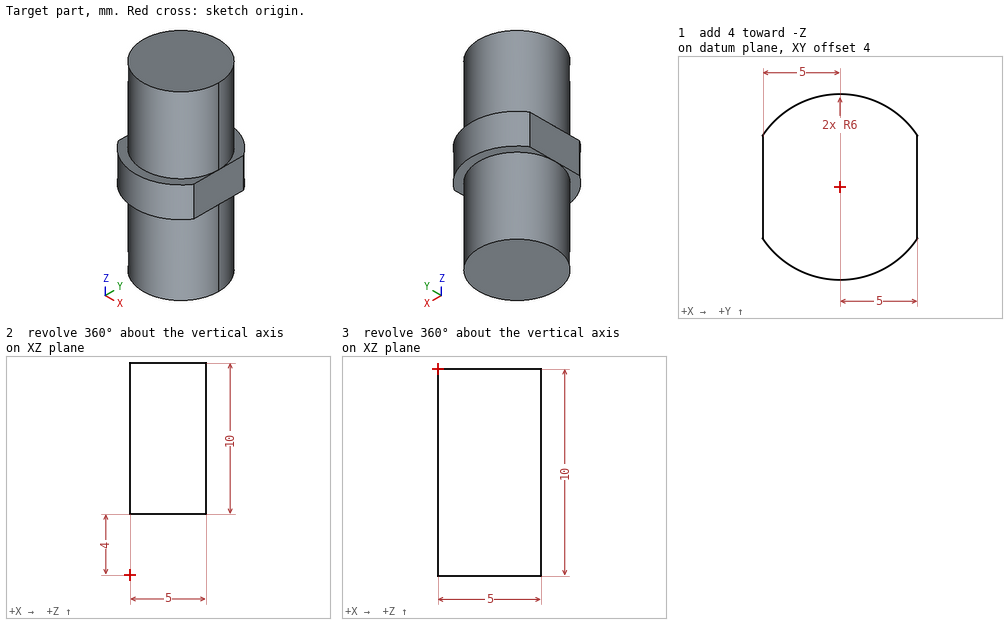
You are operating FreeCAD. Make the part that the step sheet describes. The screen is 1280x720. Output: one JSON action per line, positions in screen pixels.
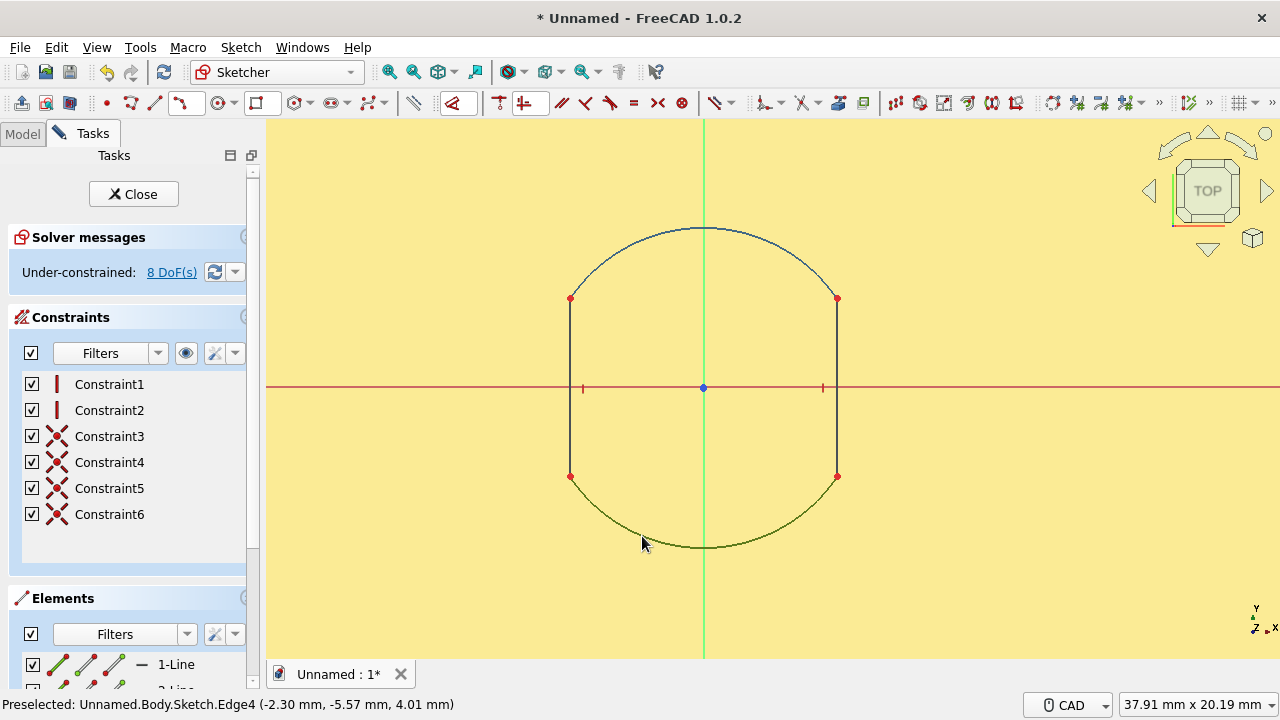
{"action": "left_click", "coordinate": [500, 104]}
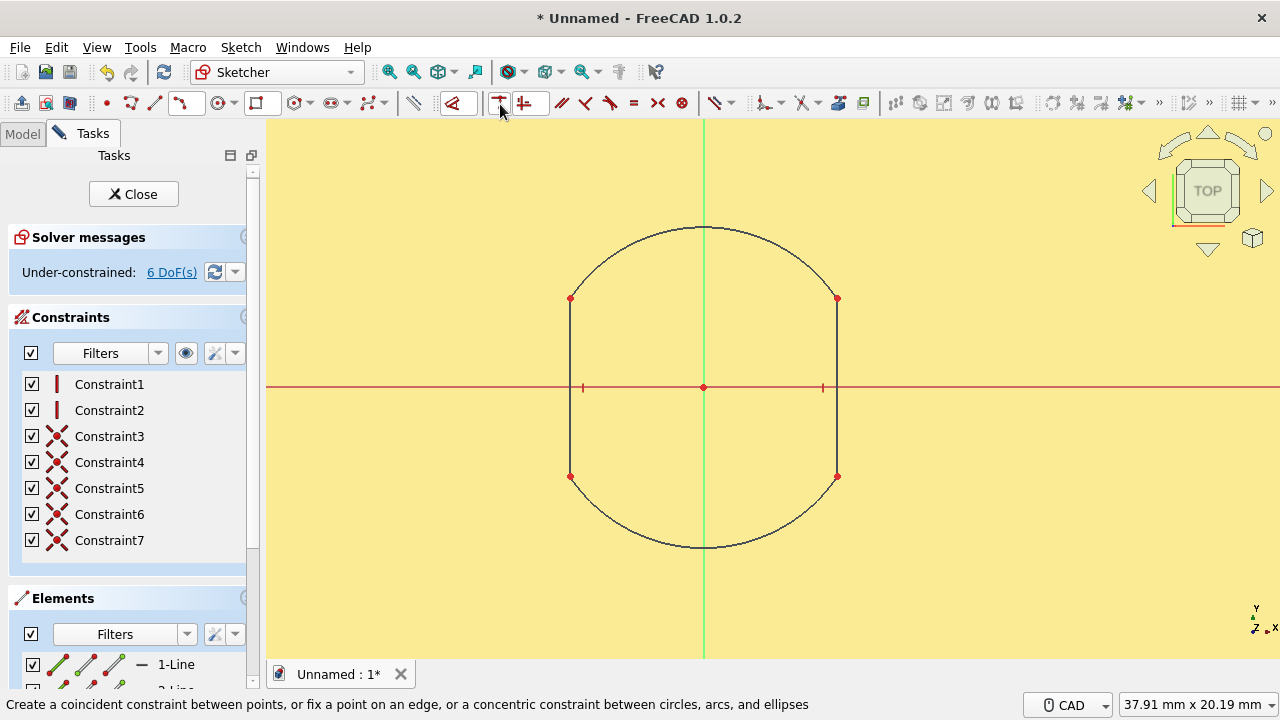
{"action": "left_click_drag", "start_coordinate": [693, 377], "coordinate": [714, 397]}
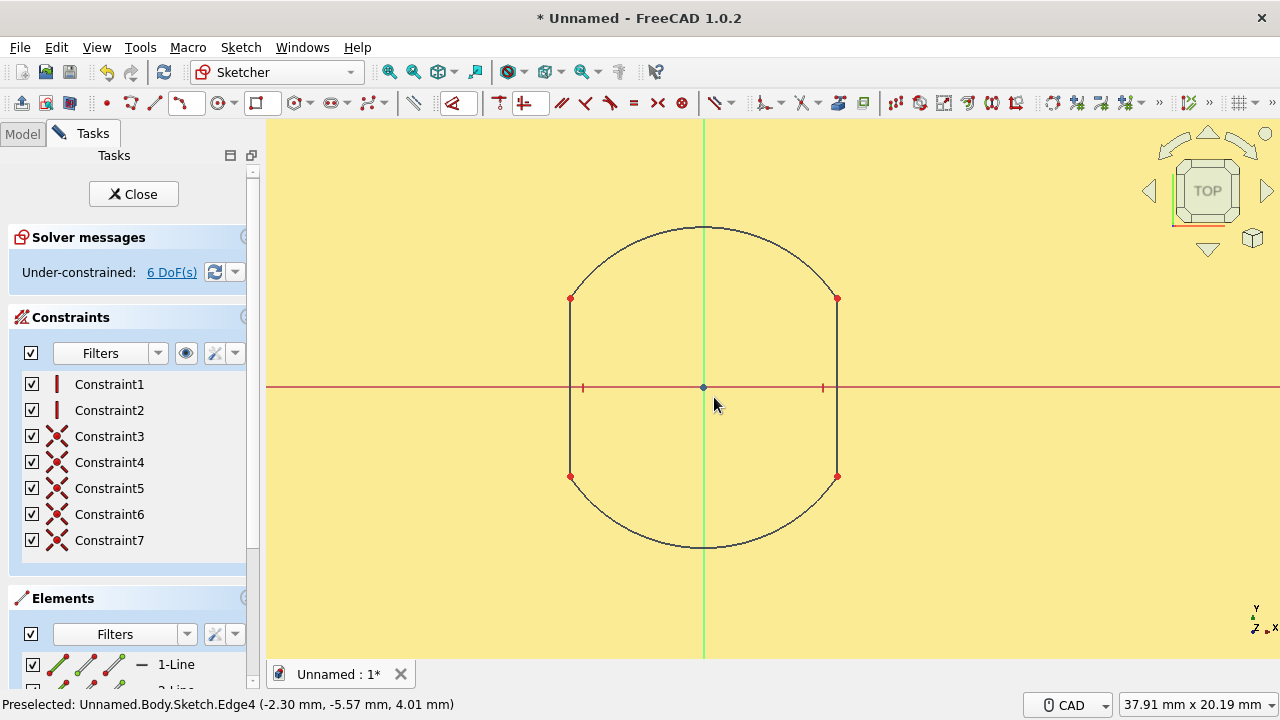
{"action": "left_click", "coordinate": [500, 104]}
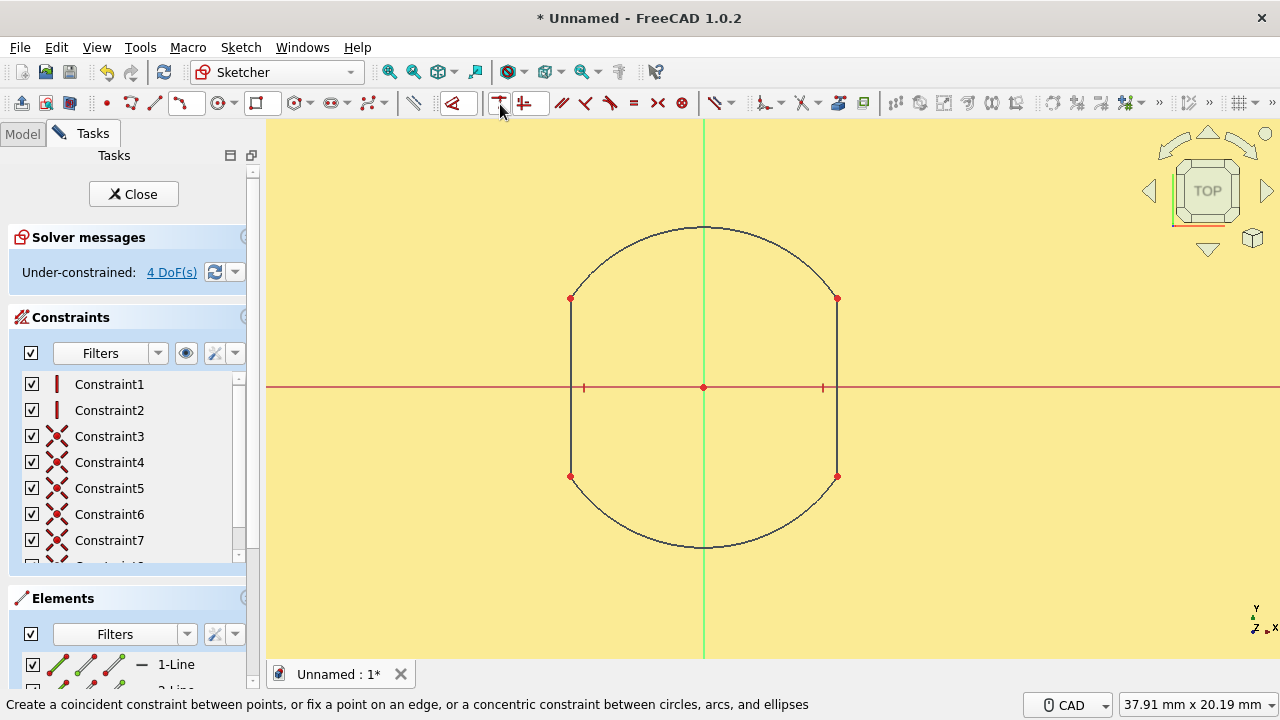
{"action": "left_click", "coordinate": [765, 240]}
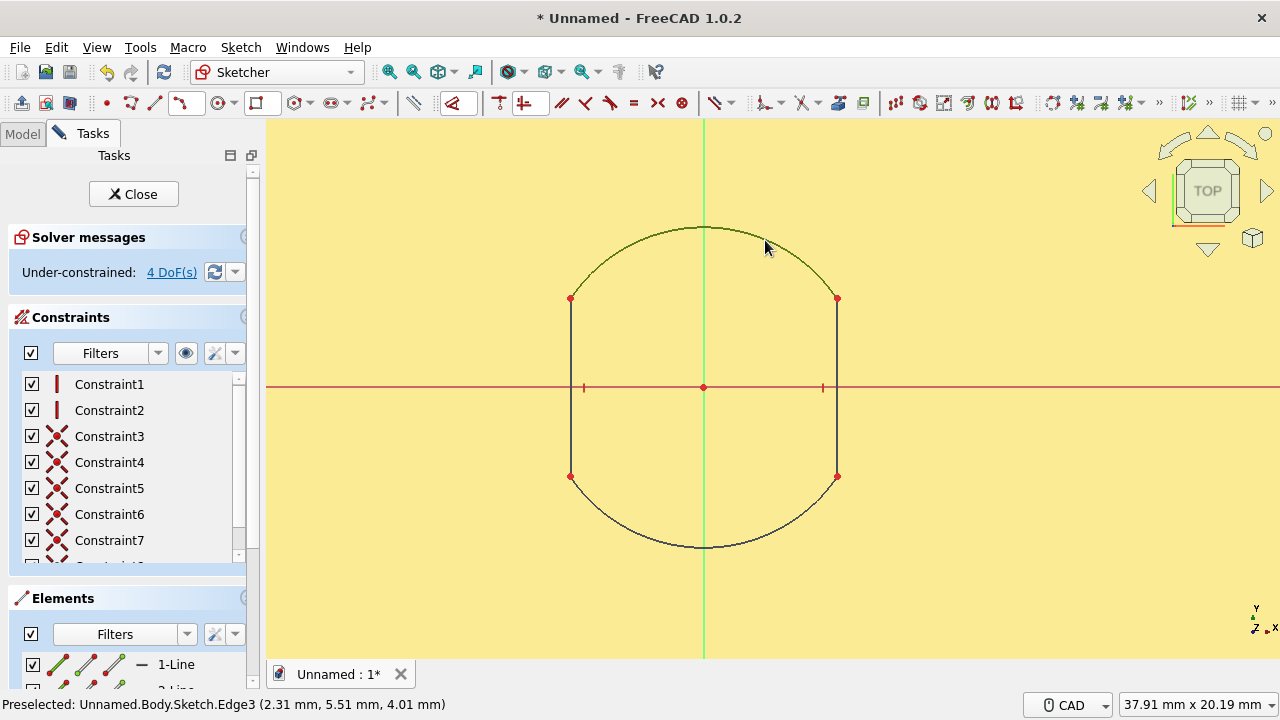
{"action": "left_click", "coordinate": [643, 536]}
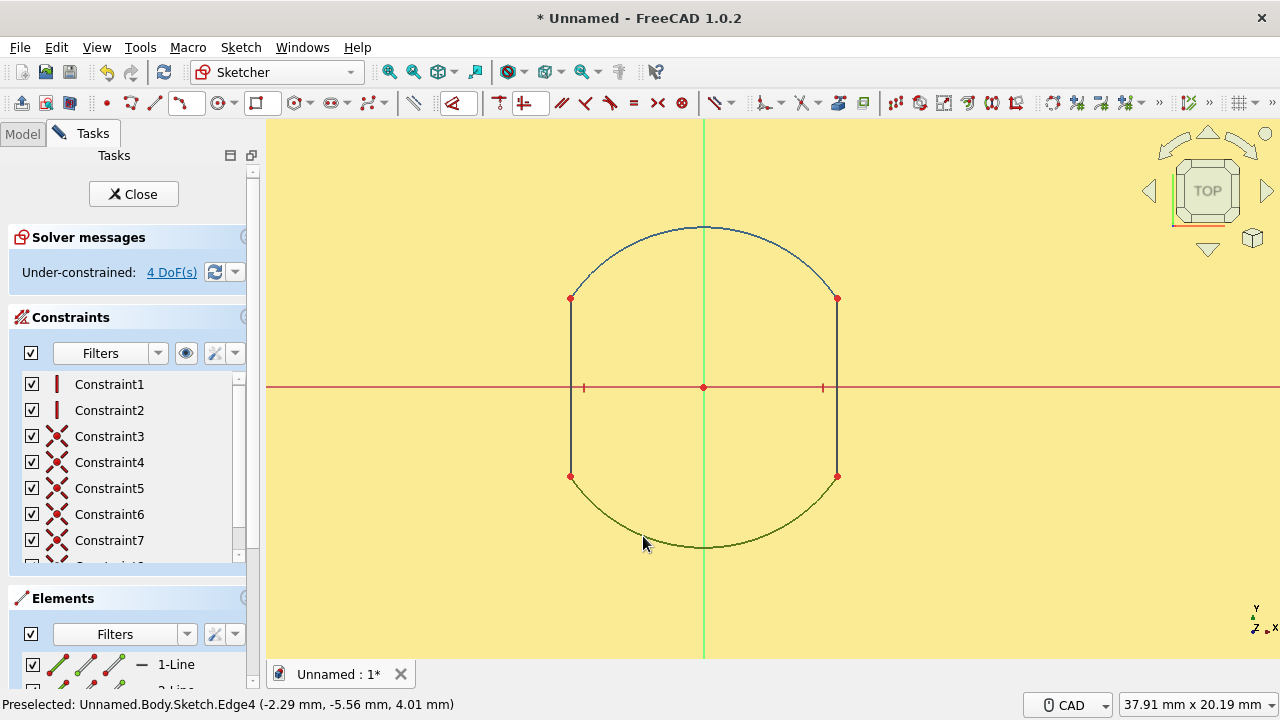
{"action": "left_click", "coordinate": [634, 104]}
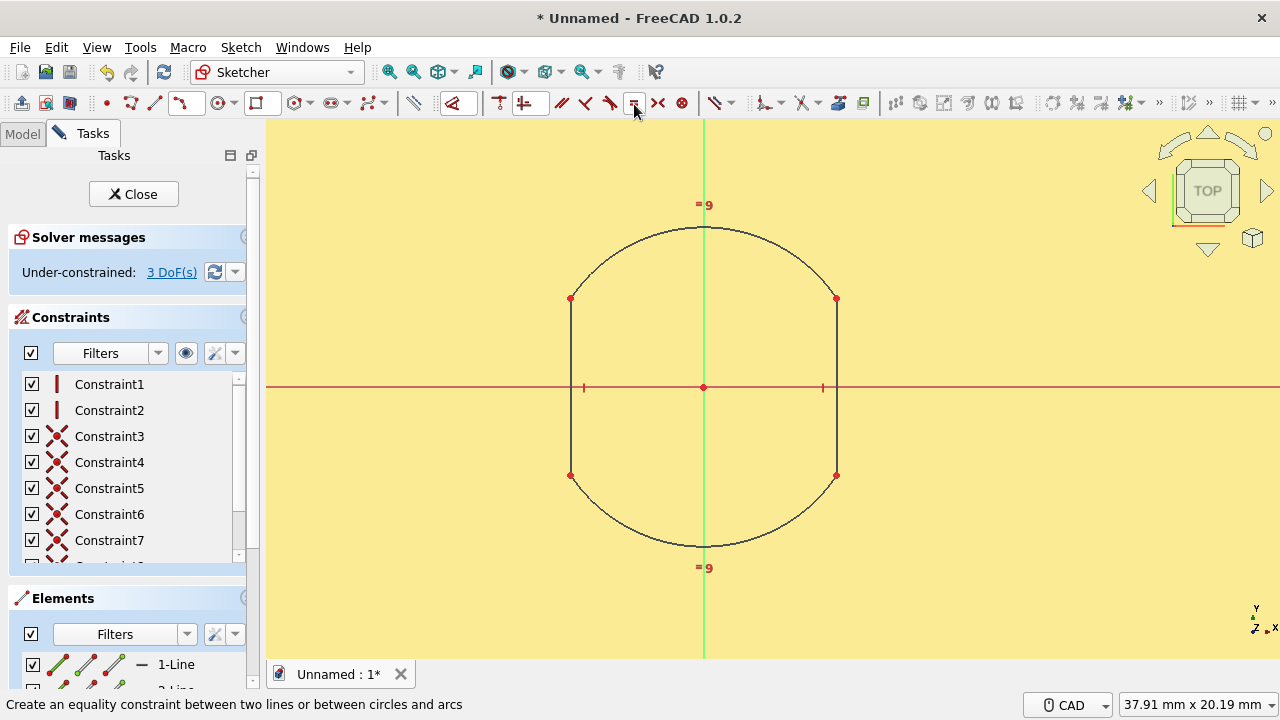
{"action": "left_click", "coordinate": [452, 104]}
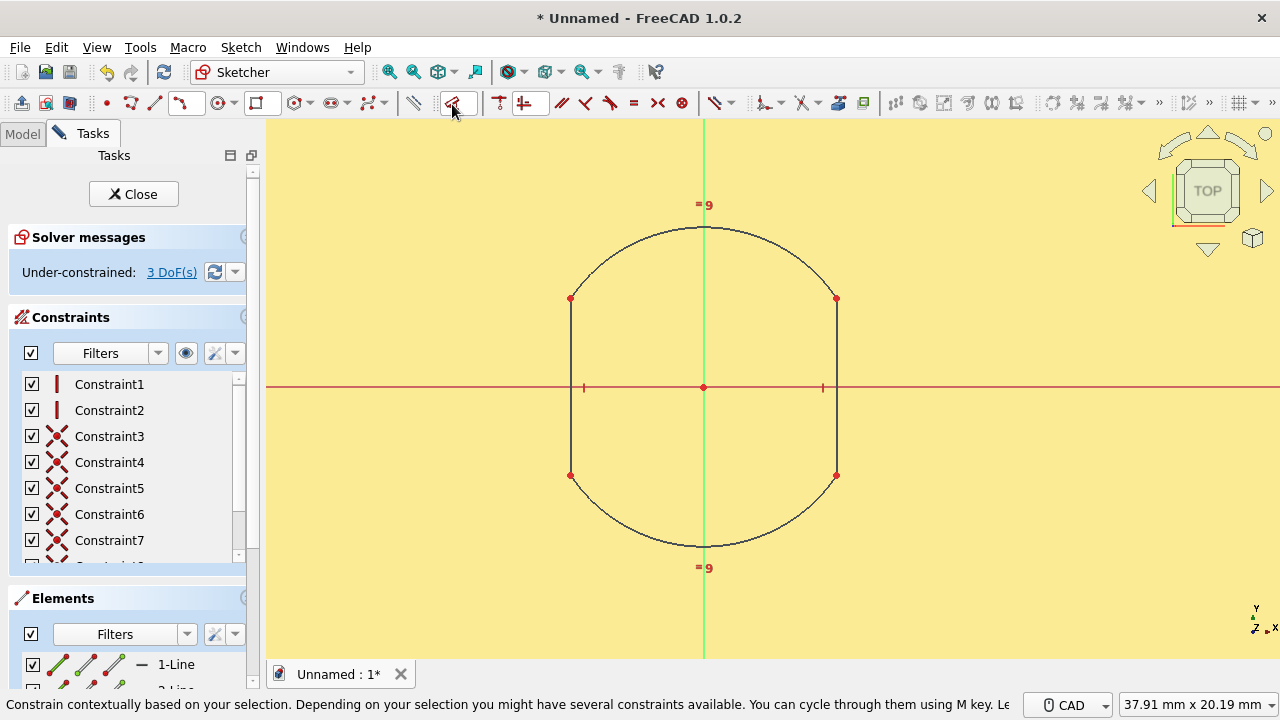
{"action": "left_click", "coordinate": [765, 240]}
{"action": "left_click", "coordinate": [777, 210]}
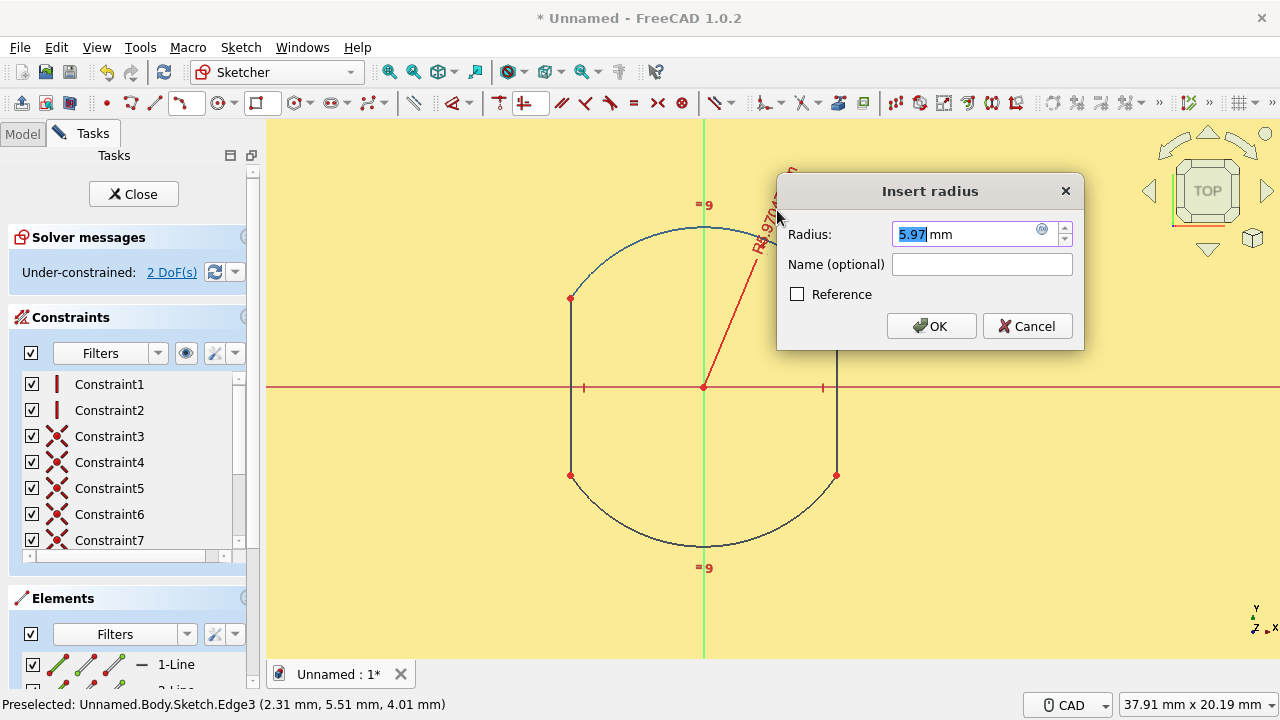
{"action": "type", "text": "6"}
{"action": "key", "text": "Return"}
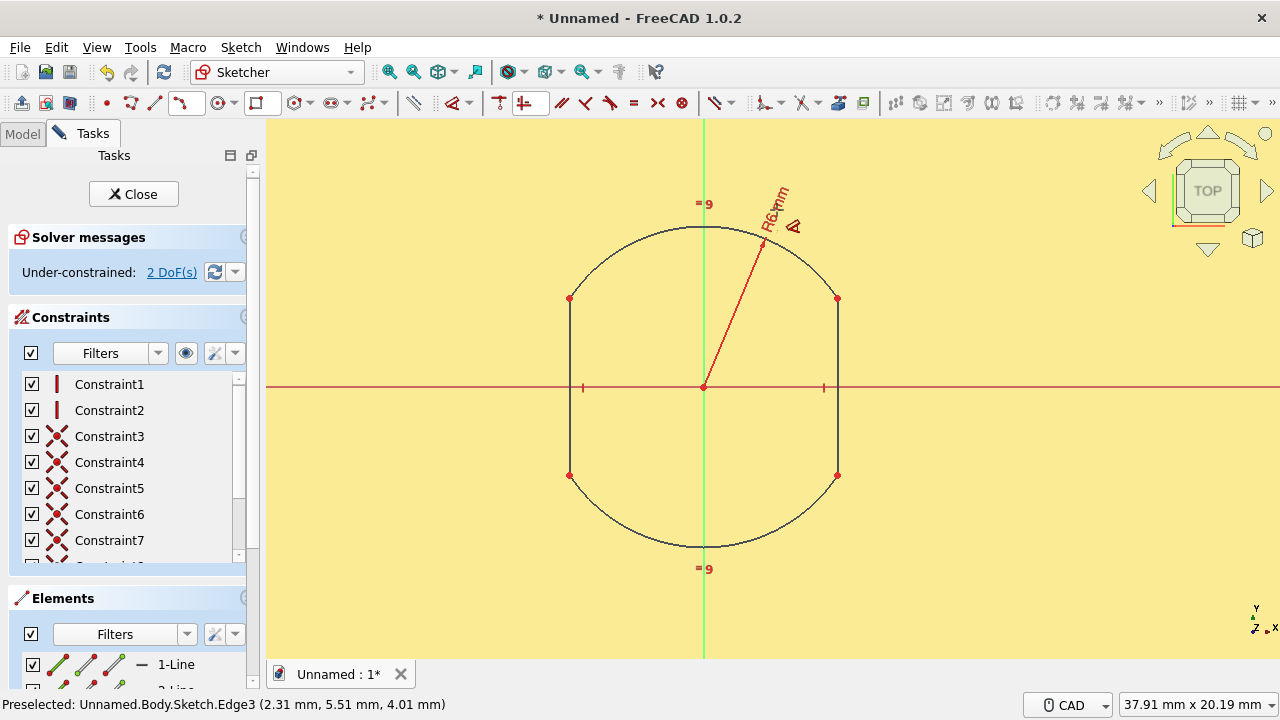
{"action": "left_click", "coordinate": [838, 475]}
{"action": "left_click", "coordinate": [771, 509]}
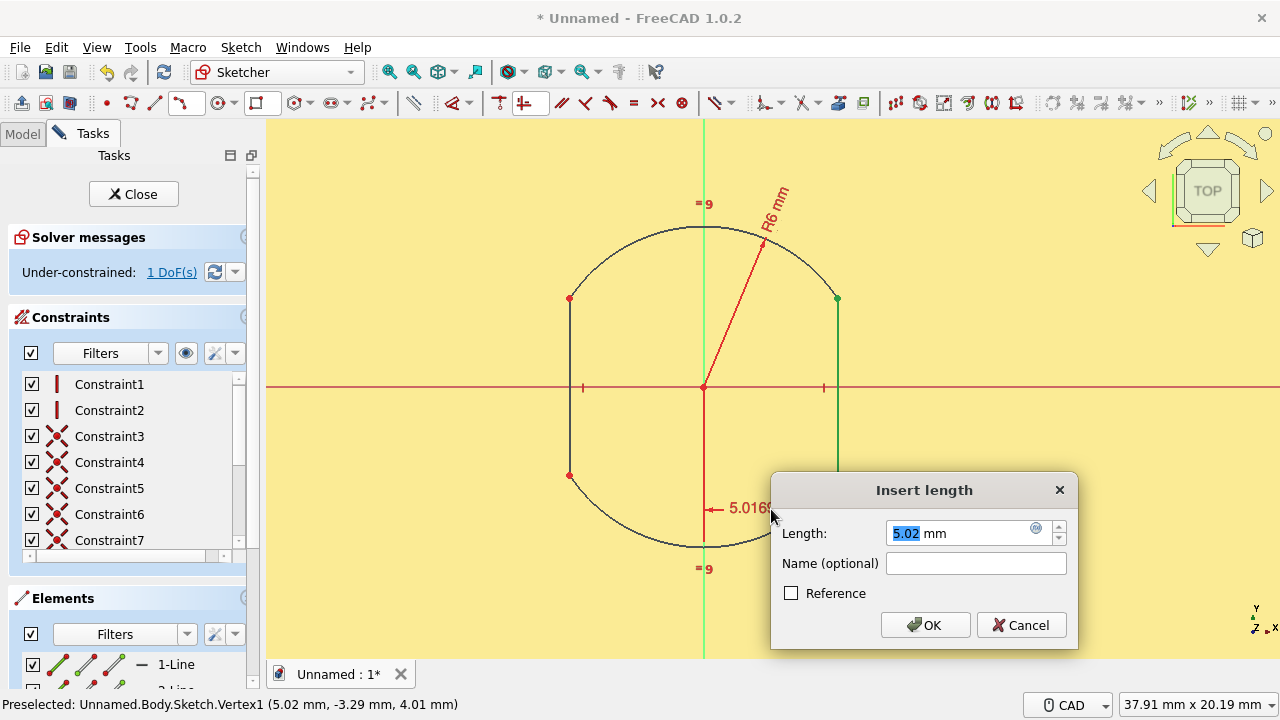
{"action": "type", "text": "5"}
{"action": "key", "text": "Return"}